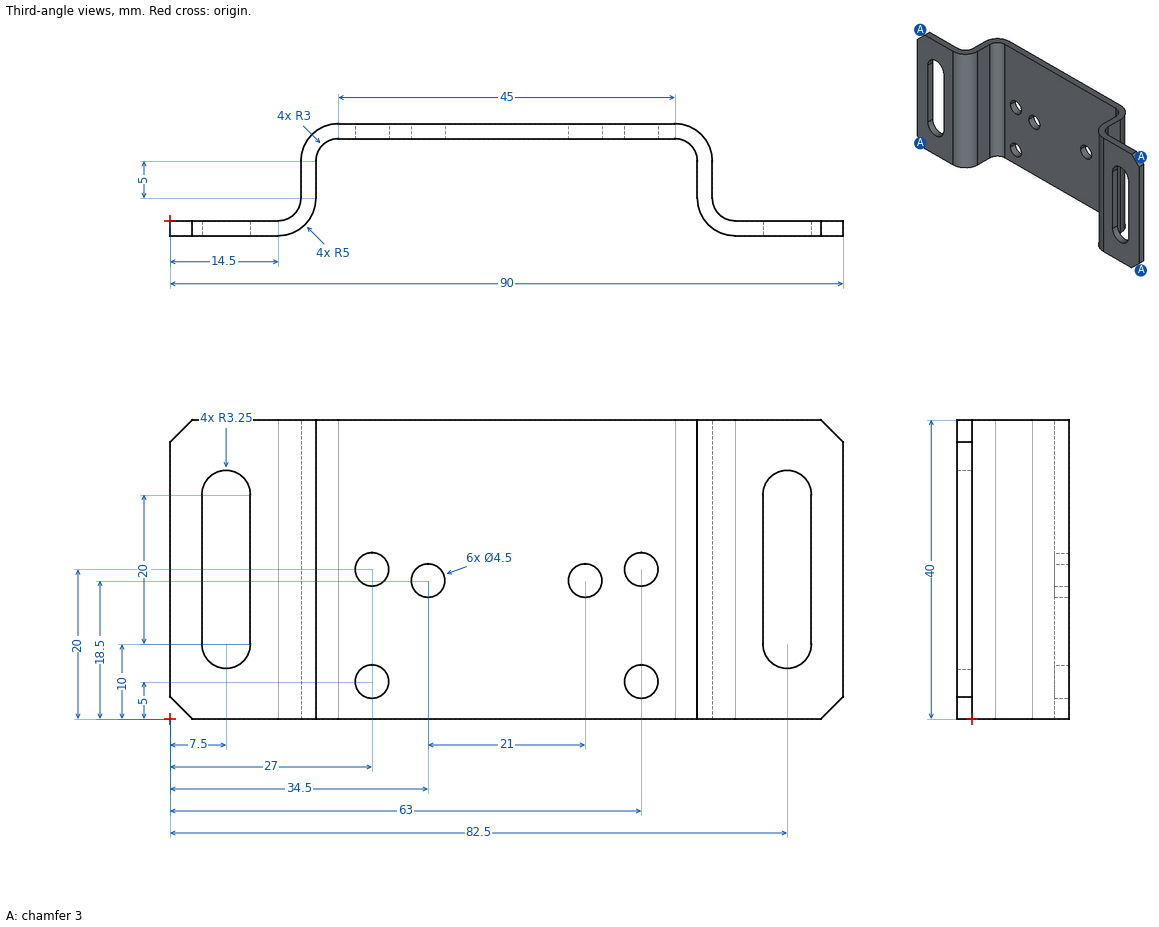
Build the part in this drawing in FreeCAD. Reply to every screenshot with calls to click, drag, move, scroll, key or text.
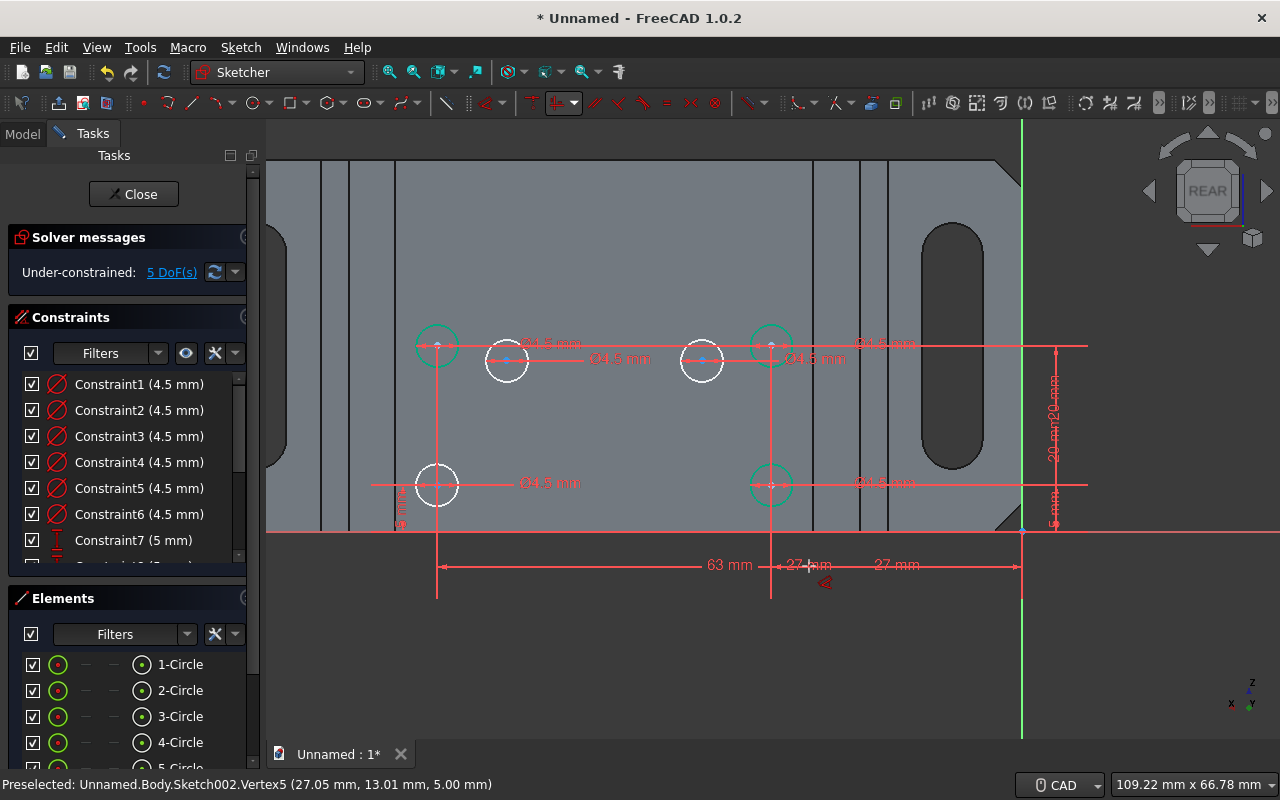
click(437, 485)
click(595, 566)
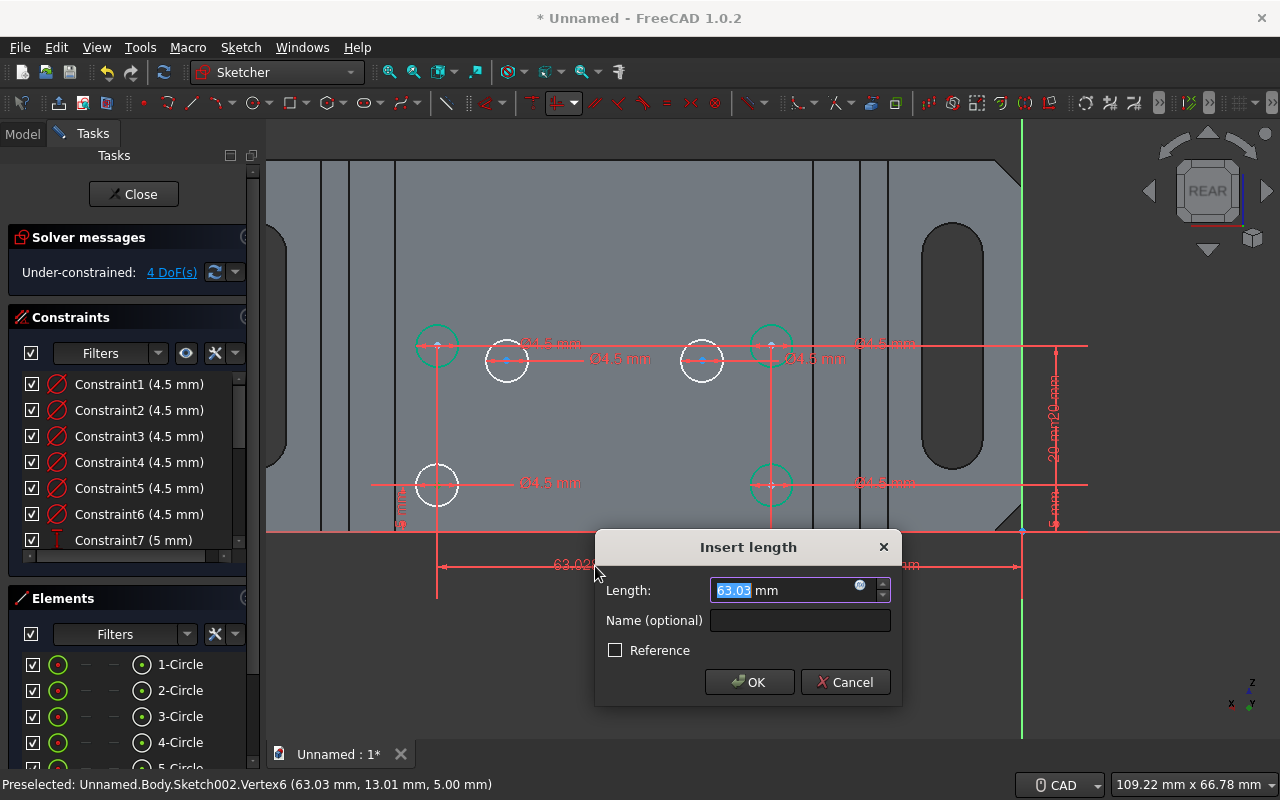
text(63)
key(Return)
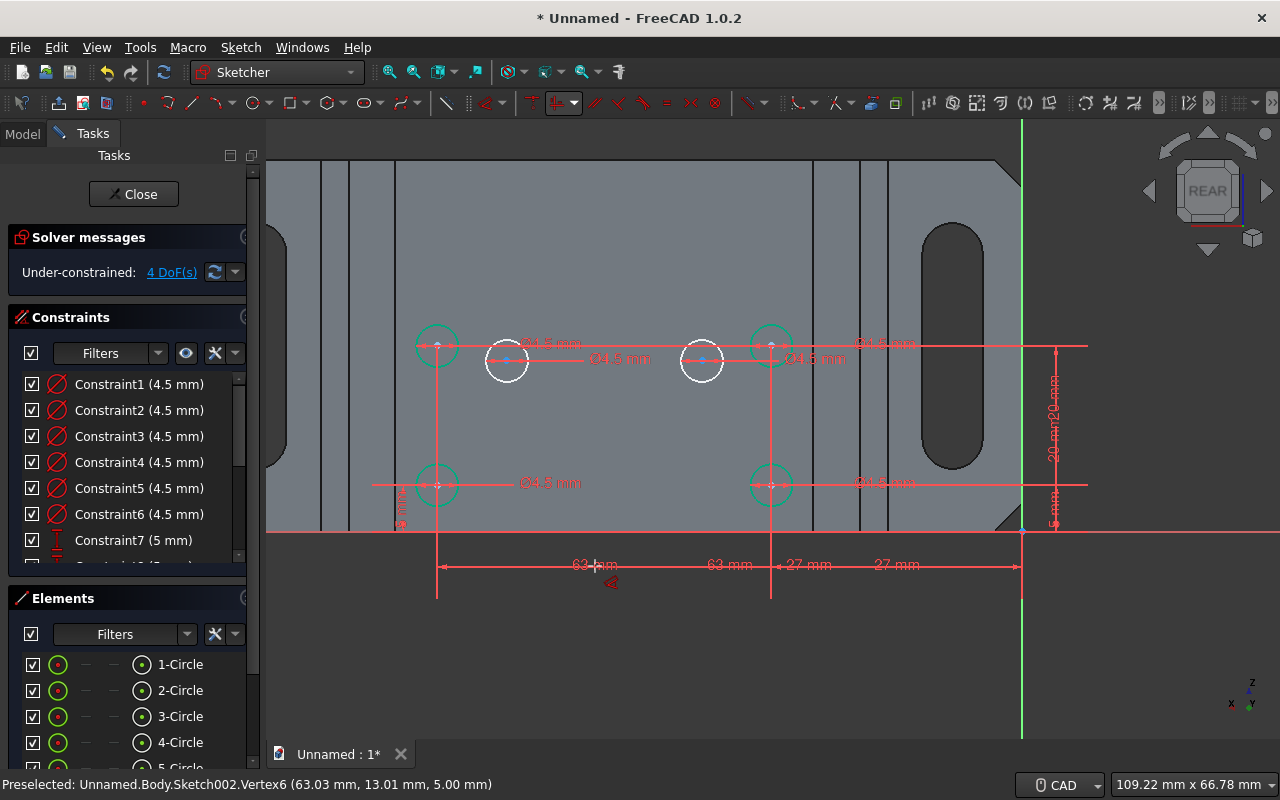
click(702, 361)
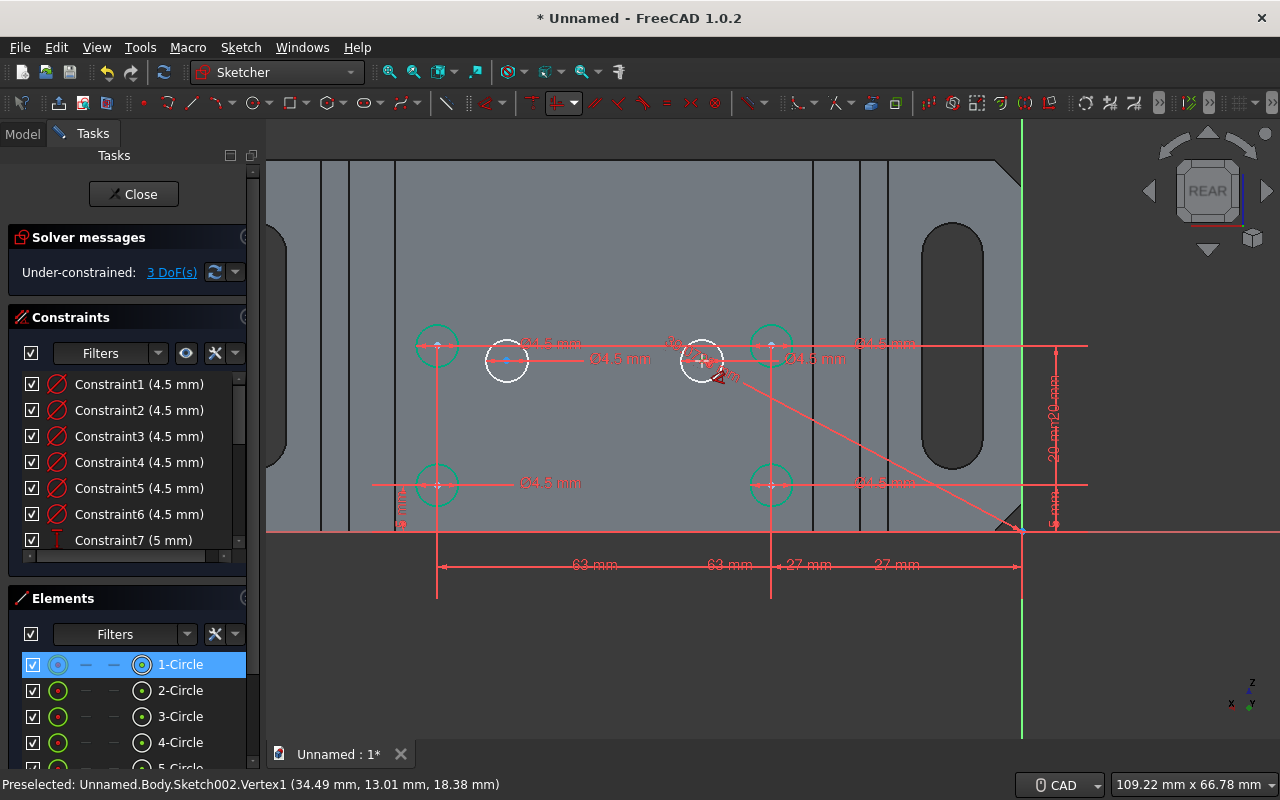
click(507, 361)
click(604, 327)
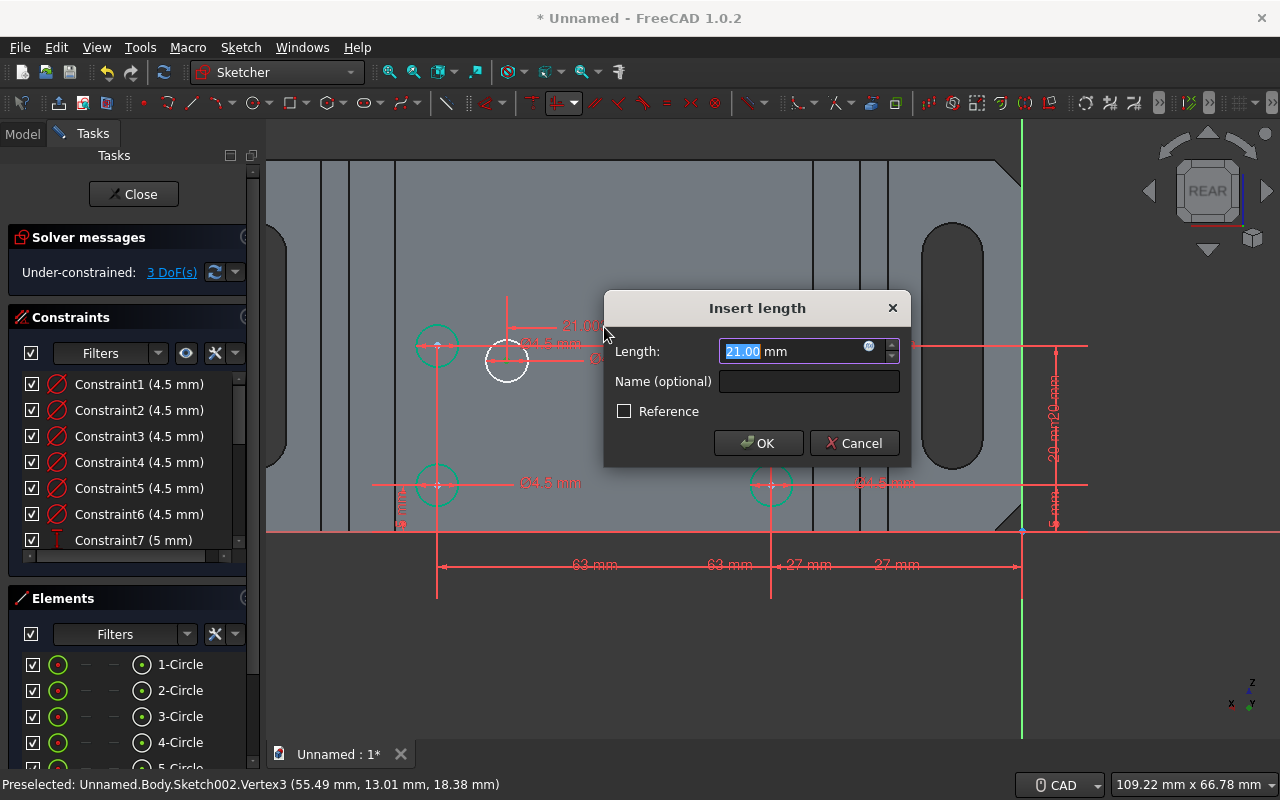
text(21)
key(Return)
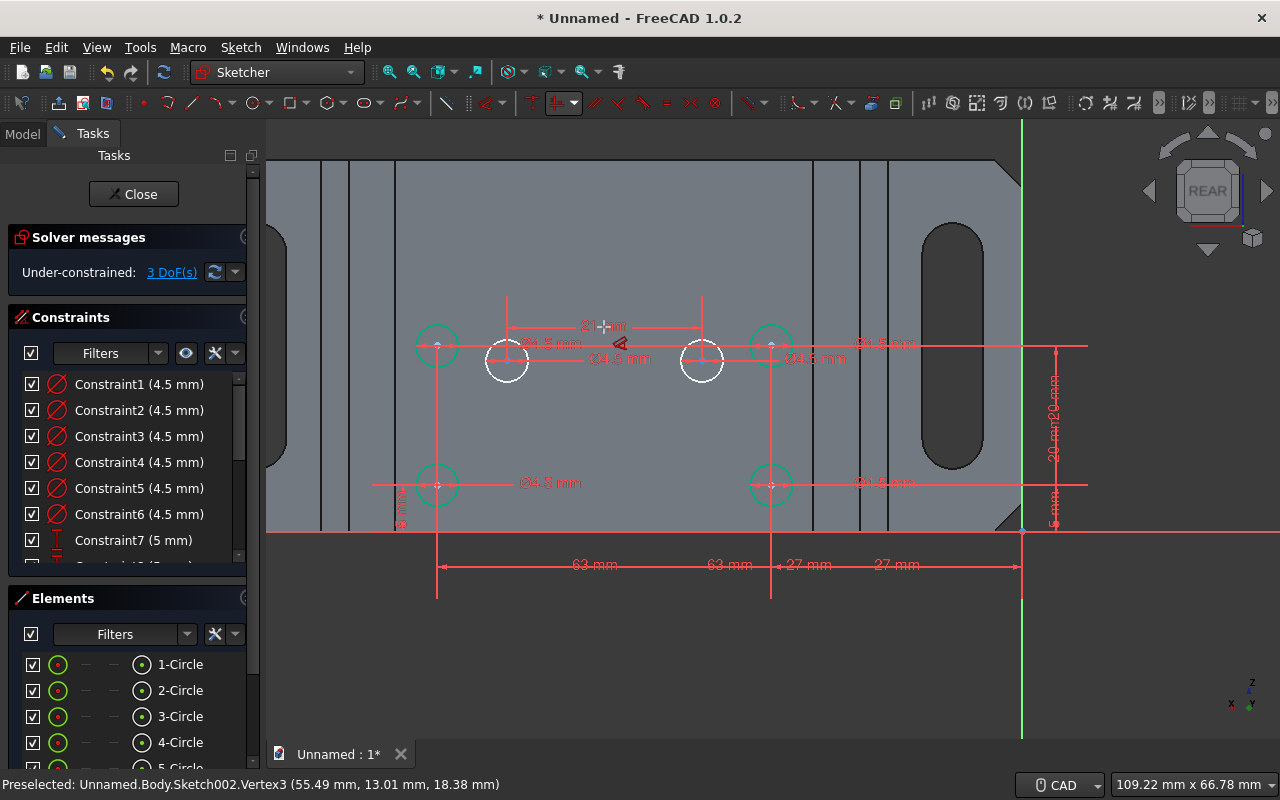
click(702, 361)
click(974, 566)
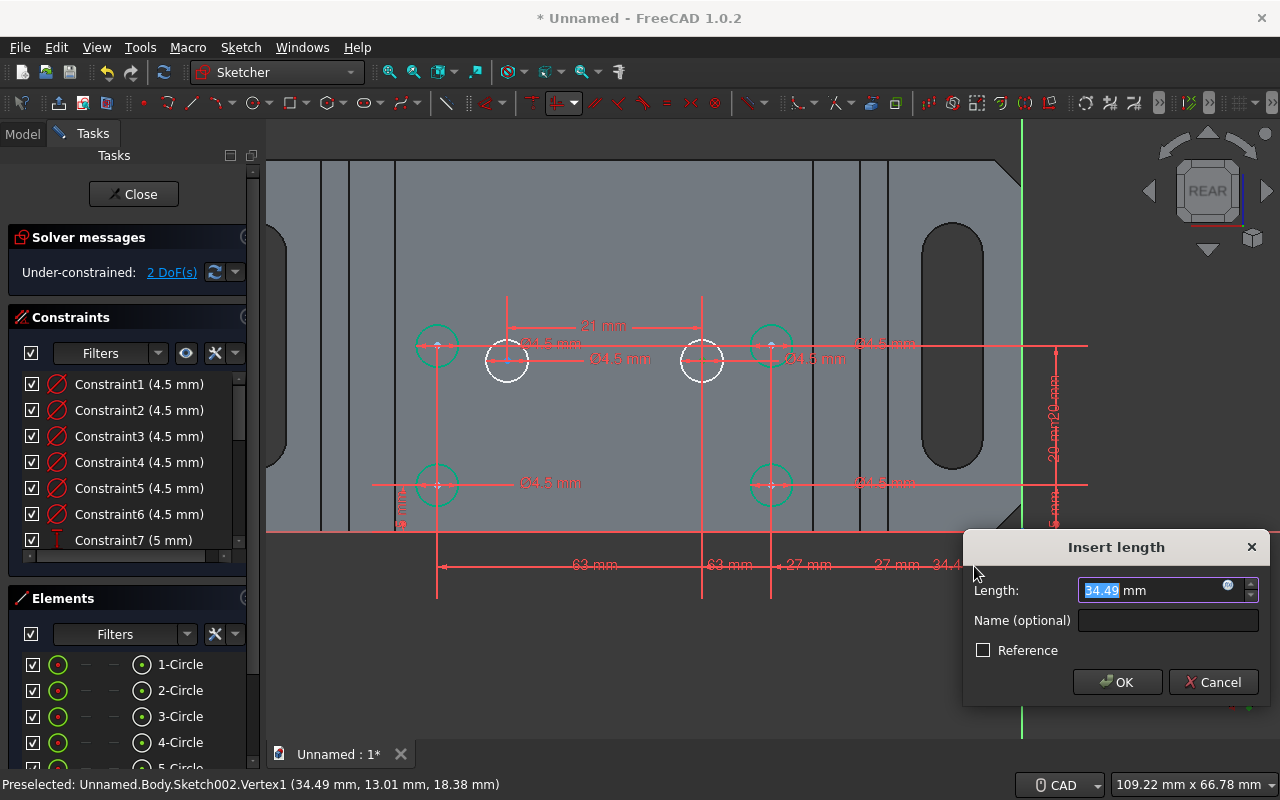
text(34.5)
key(Return)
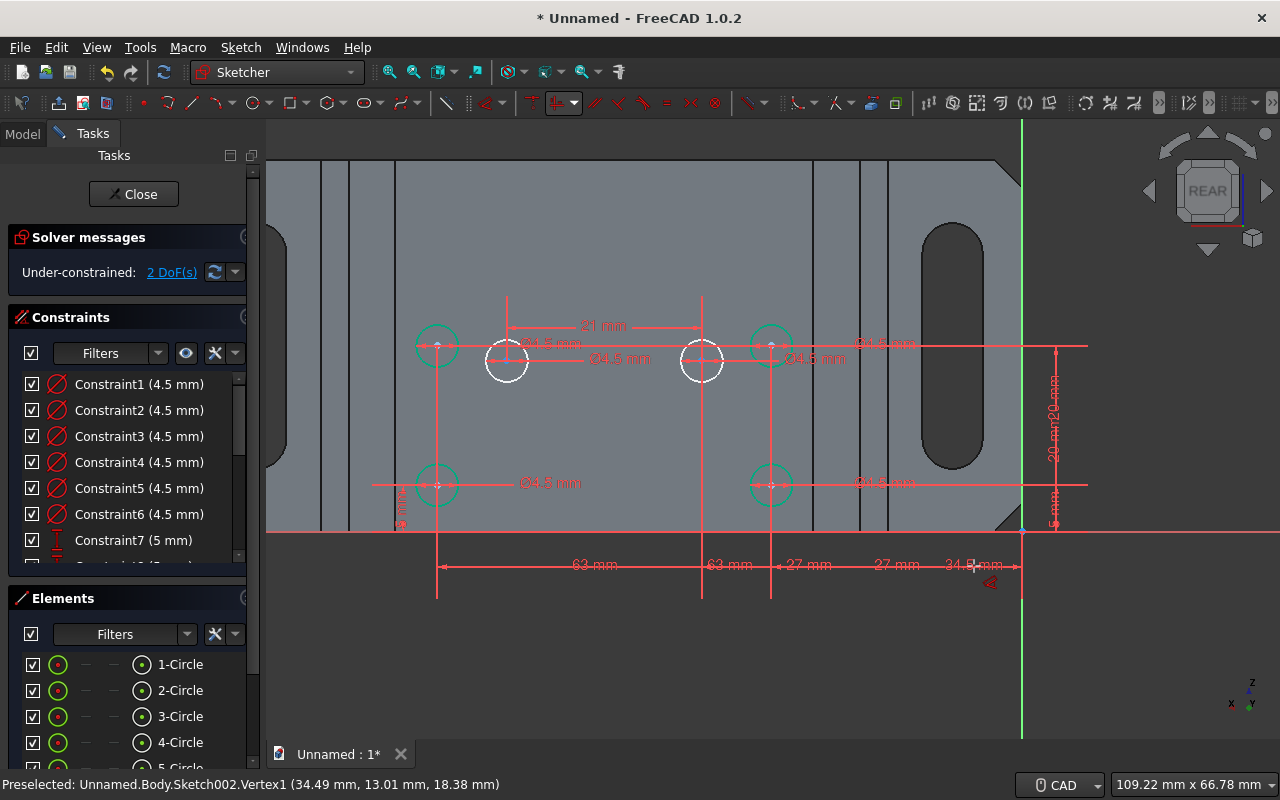
click(702, 361)
click(1056, 486)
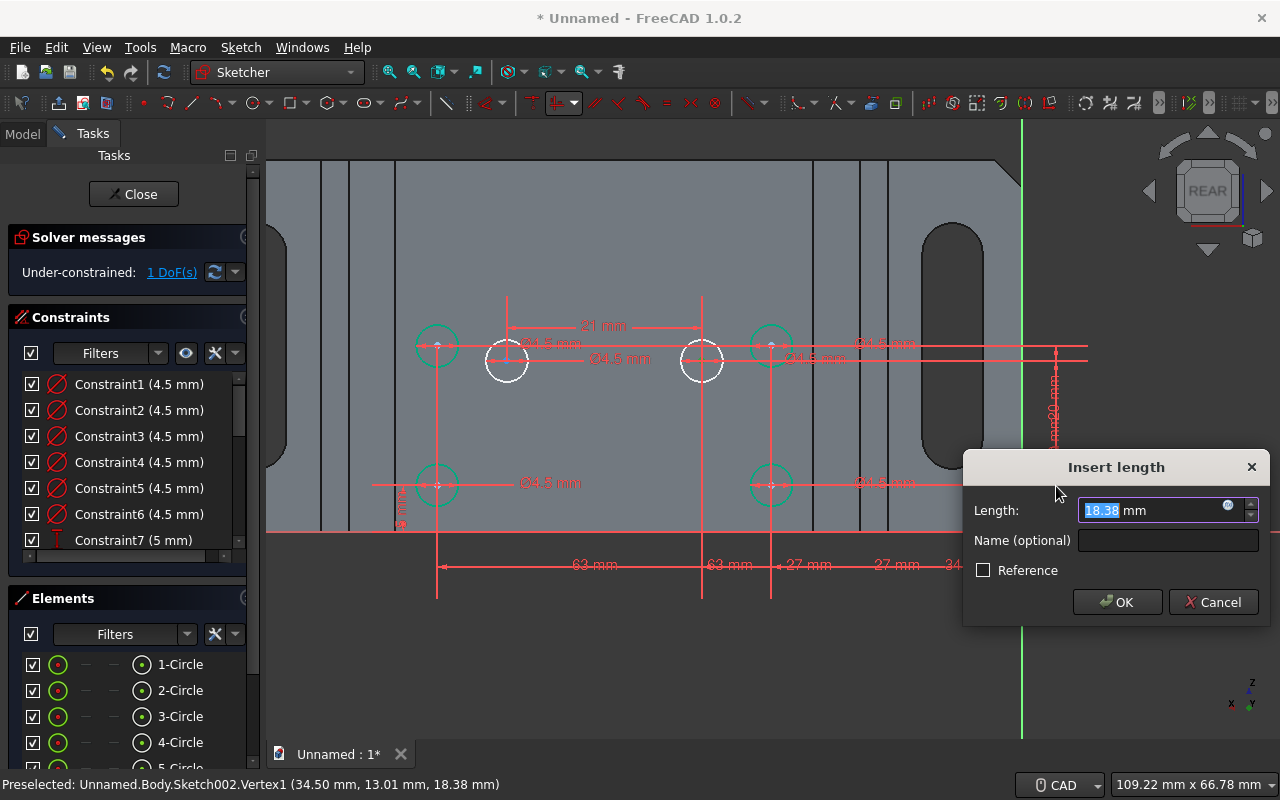
text(18.5)
key(Return)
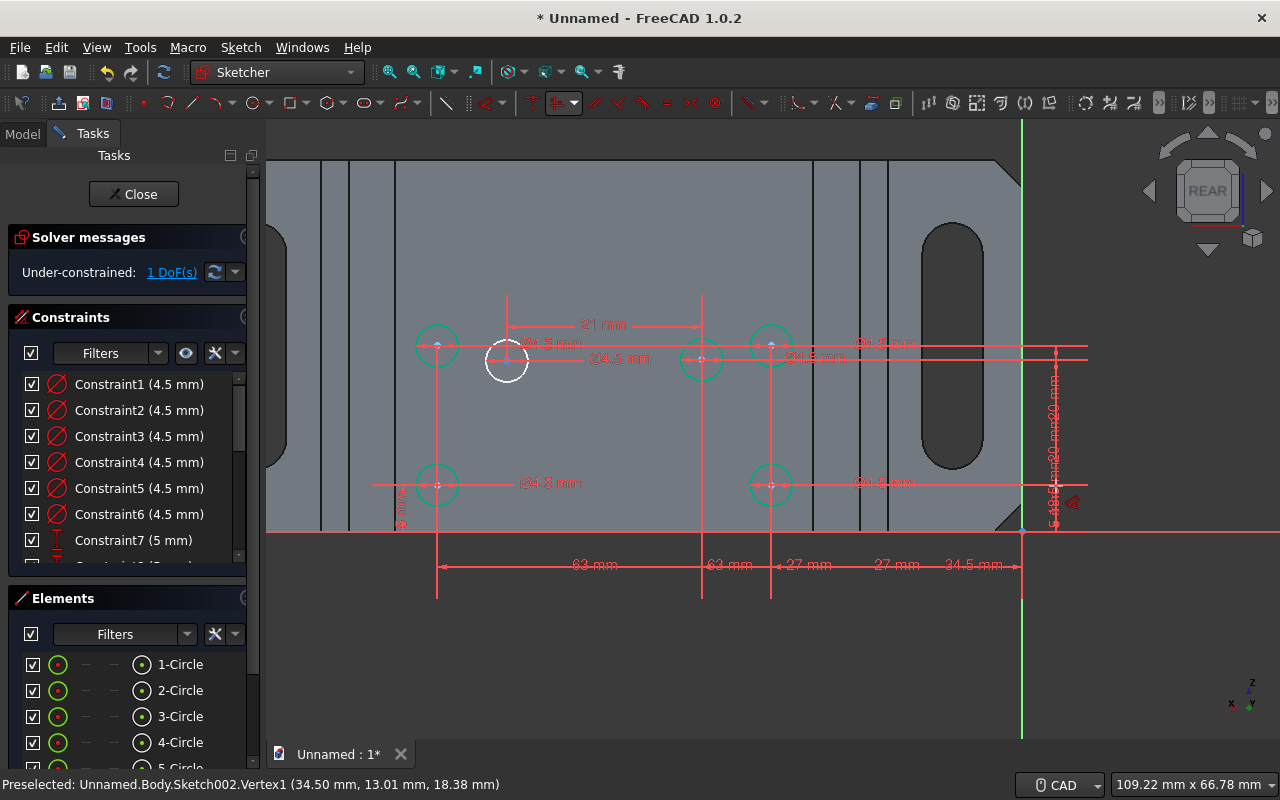
click(507, 361)
click(473, 446)